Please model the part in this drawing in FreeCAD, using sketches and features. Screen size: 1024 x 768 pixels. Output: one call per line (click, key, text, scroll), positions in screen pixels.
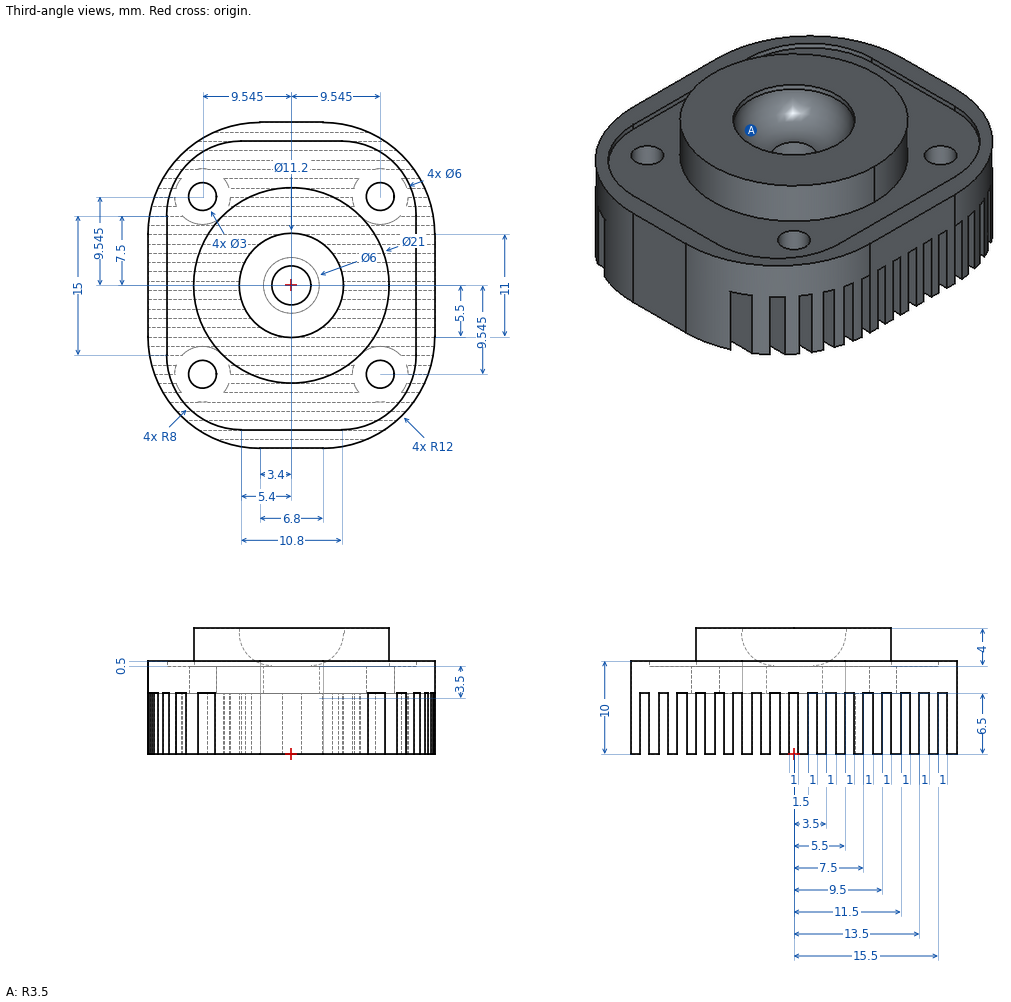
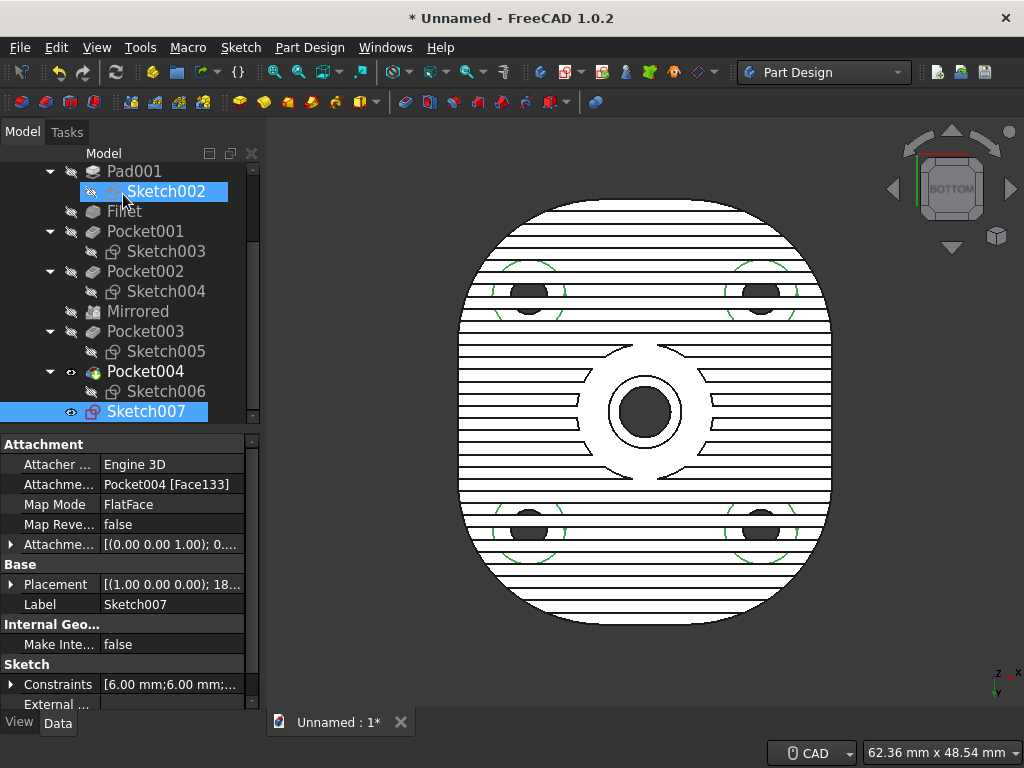
click(406, 102)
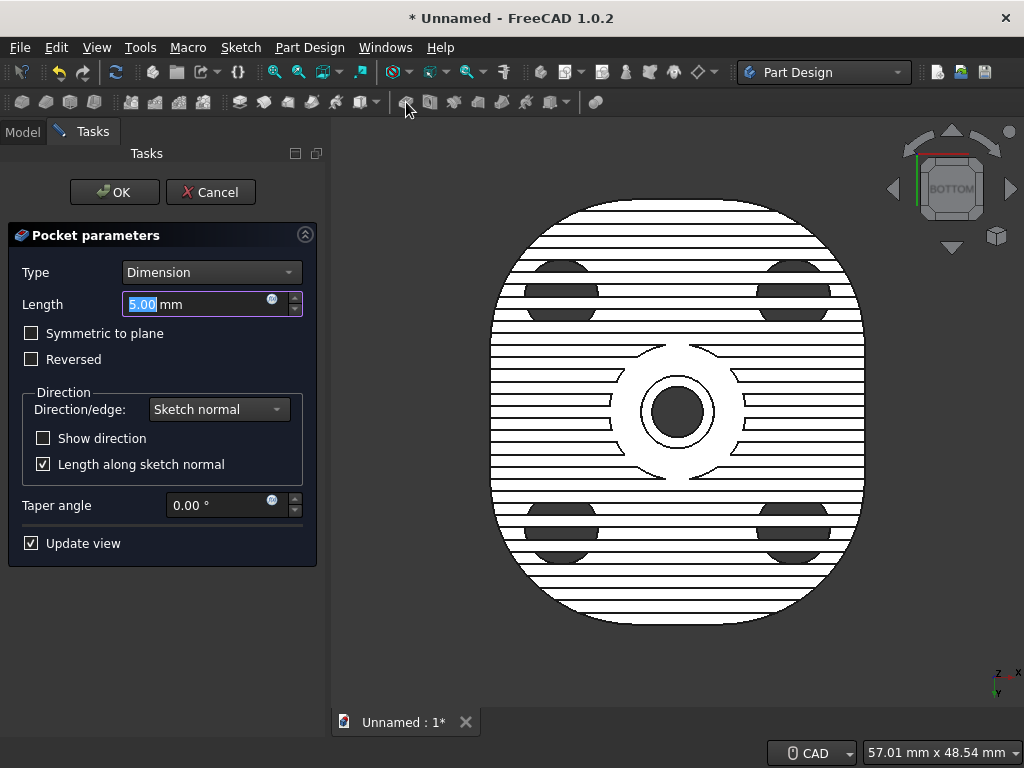
click(212, 272)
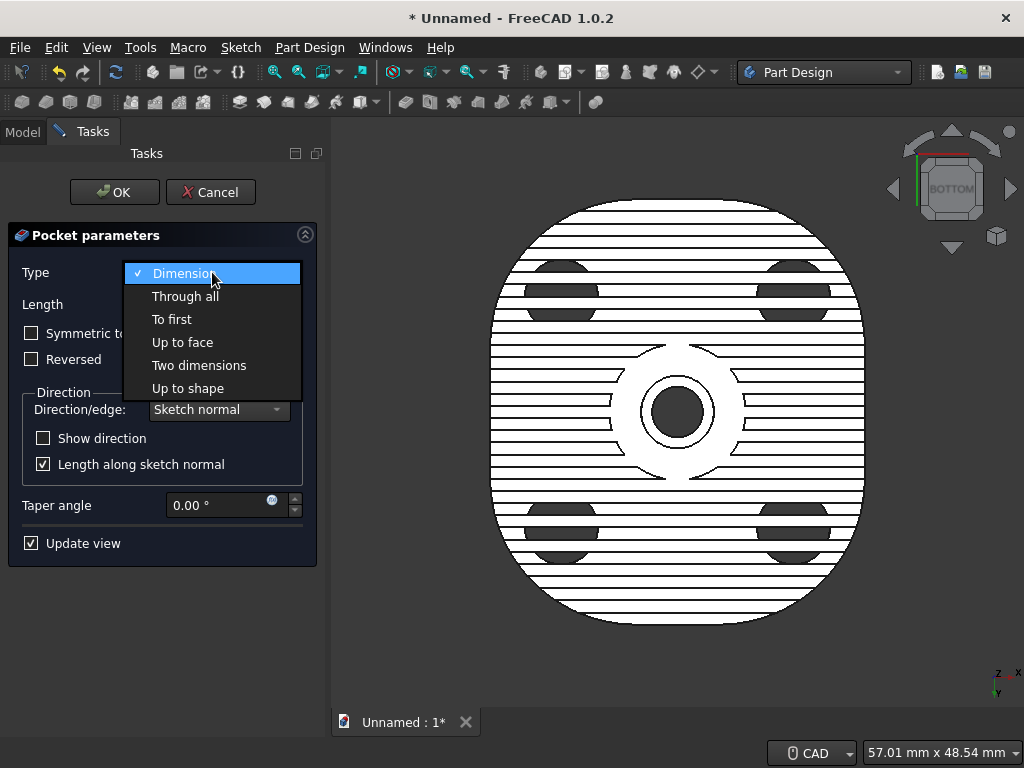
click(212, 296)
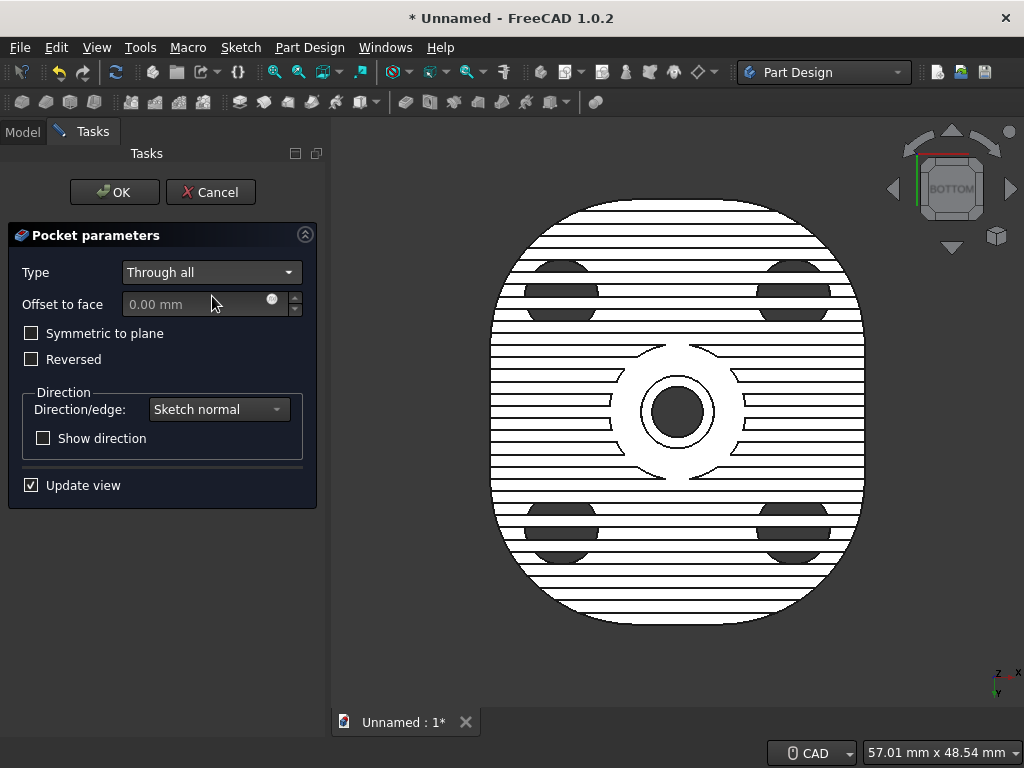
click(30, 359)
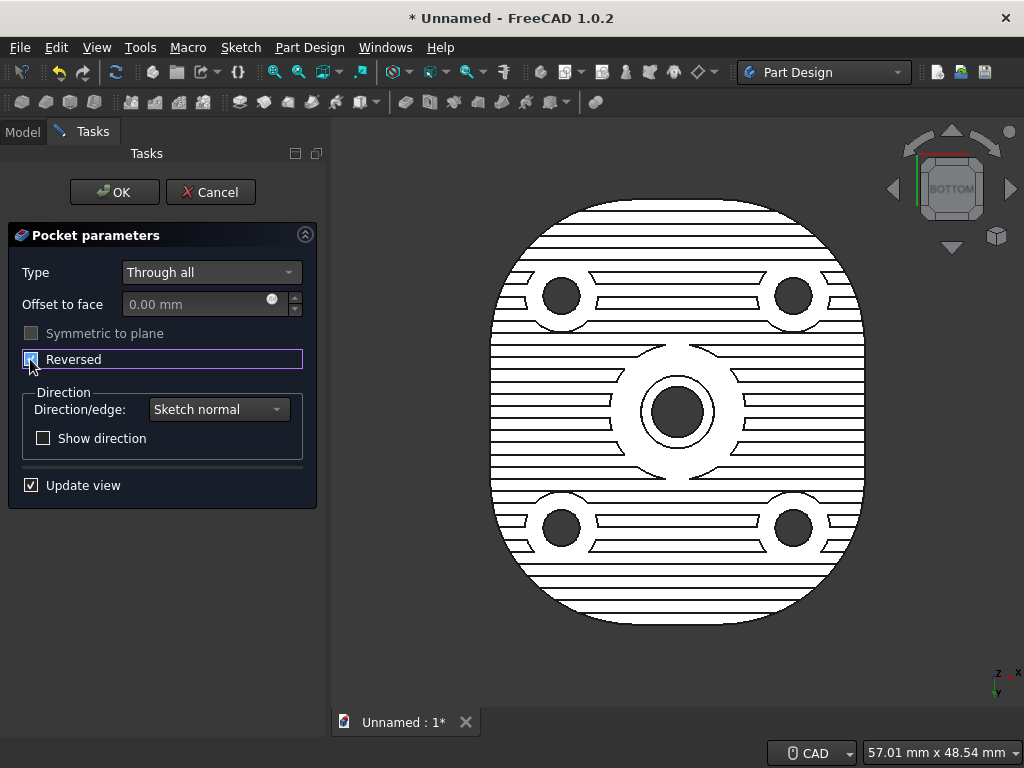
click(115, 192)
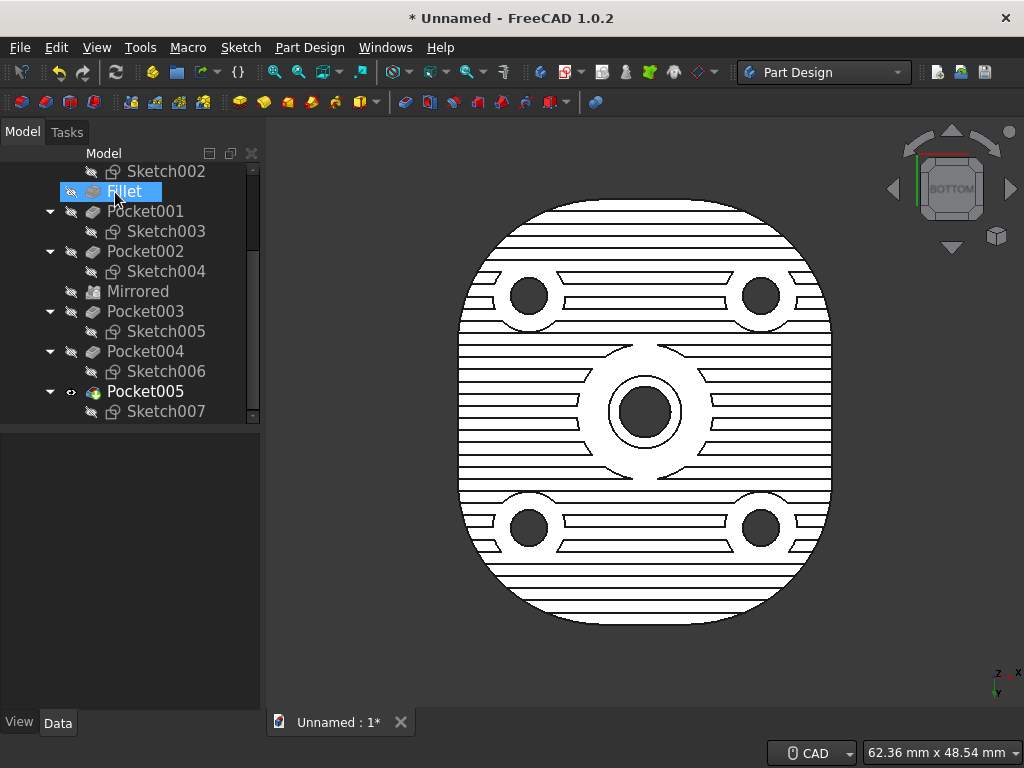
key(0)